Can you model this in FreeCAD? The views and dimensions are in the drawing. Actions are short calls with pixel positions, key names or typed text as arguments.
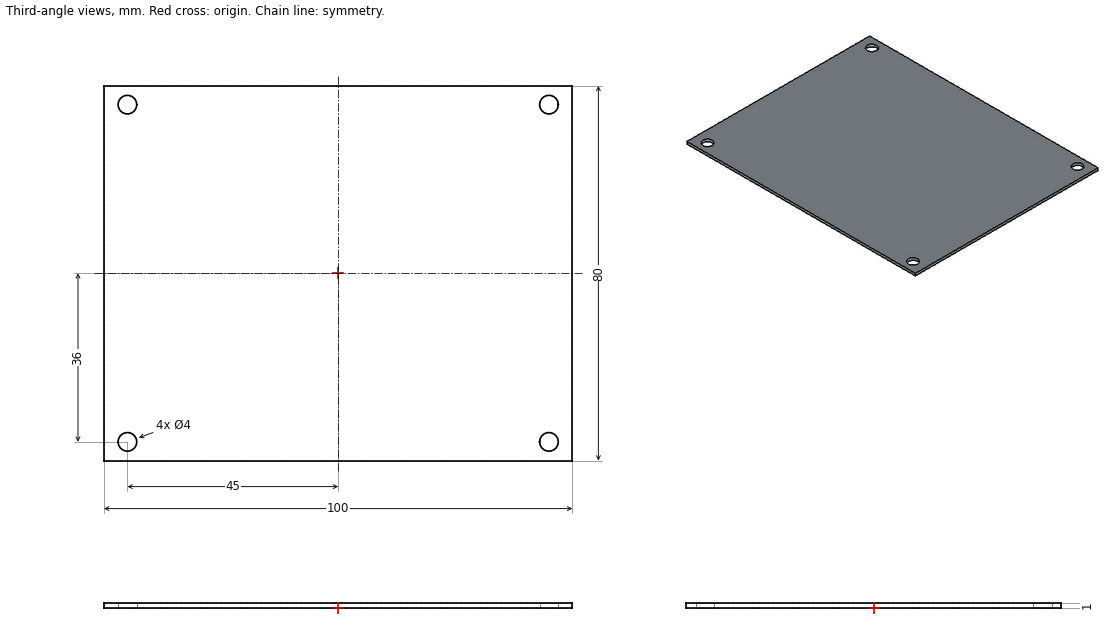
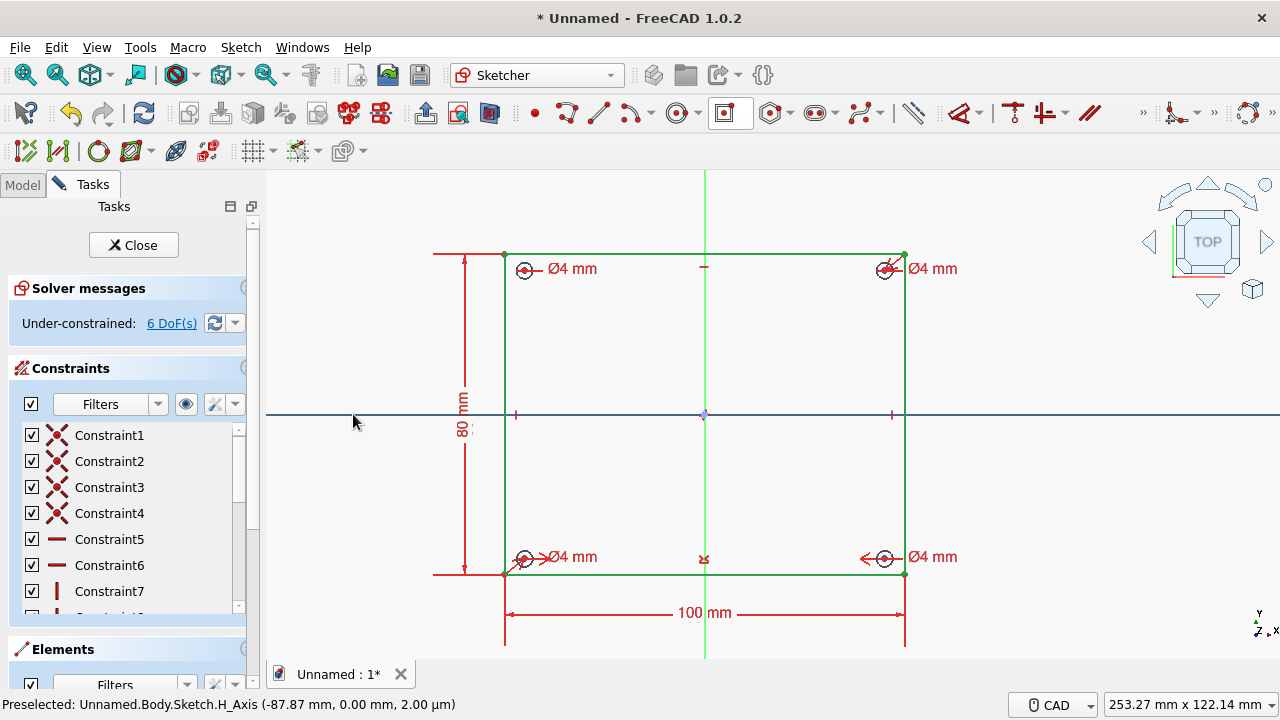
key(s)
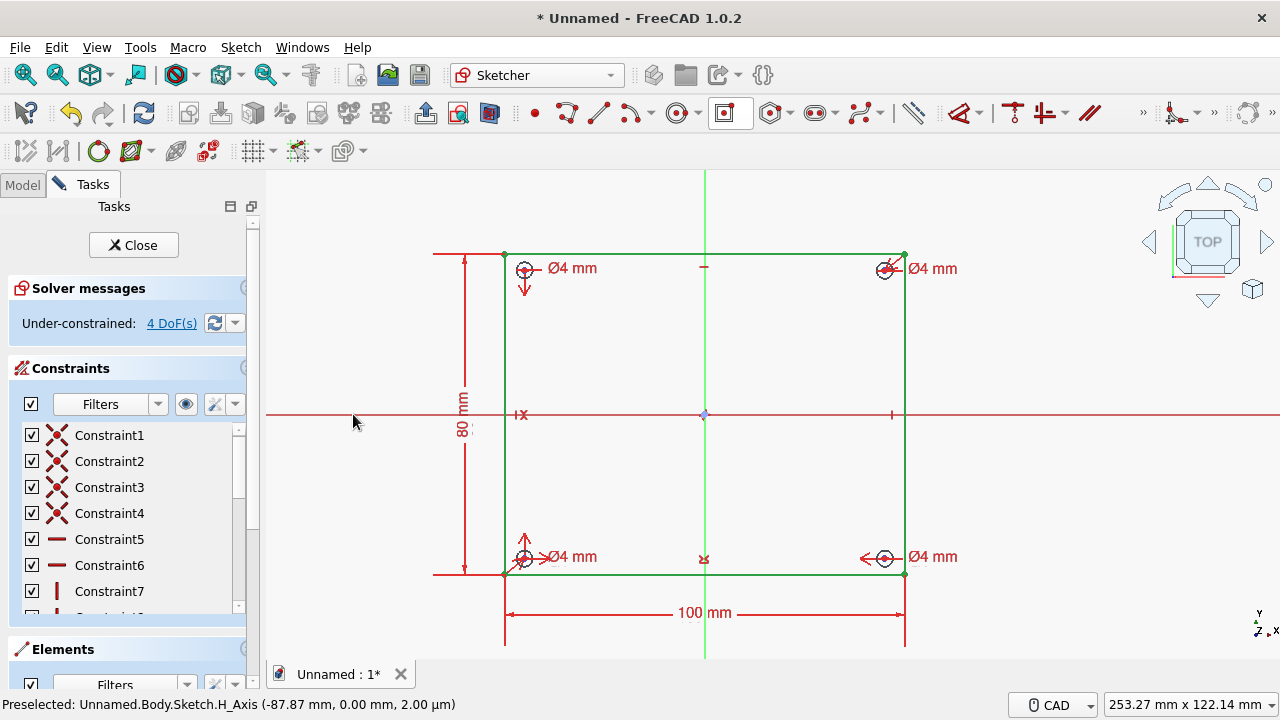
click(885, 559)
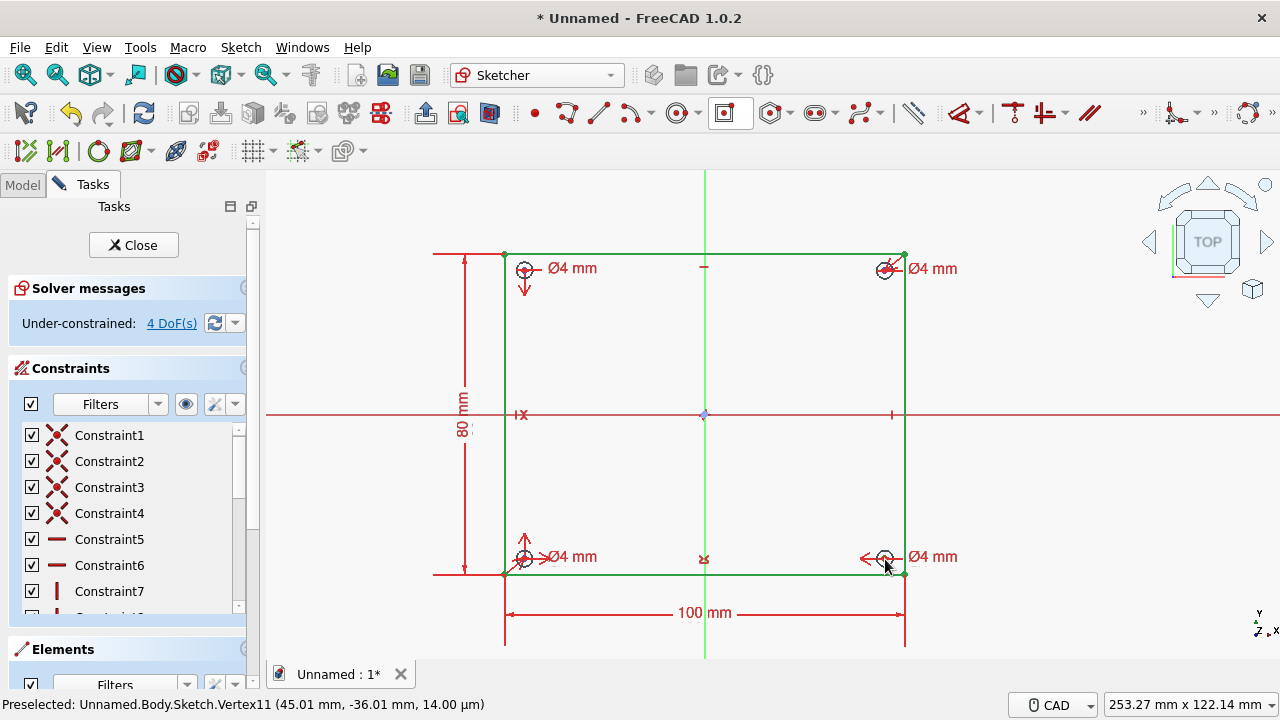
click(885, 271)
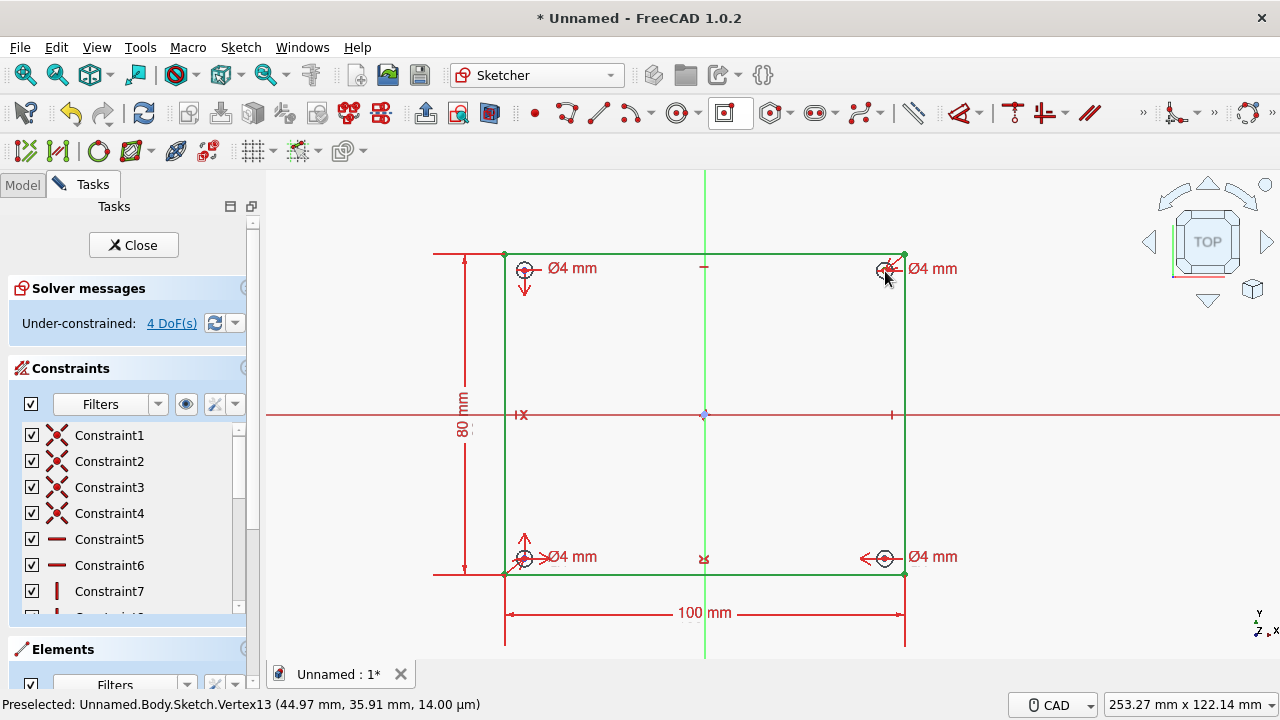
click(353, 414)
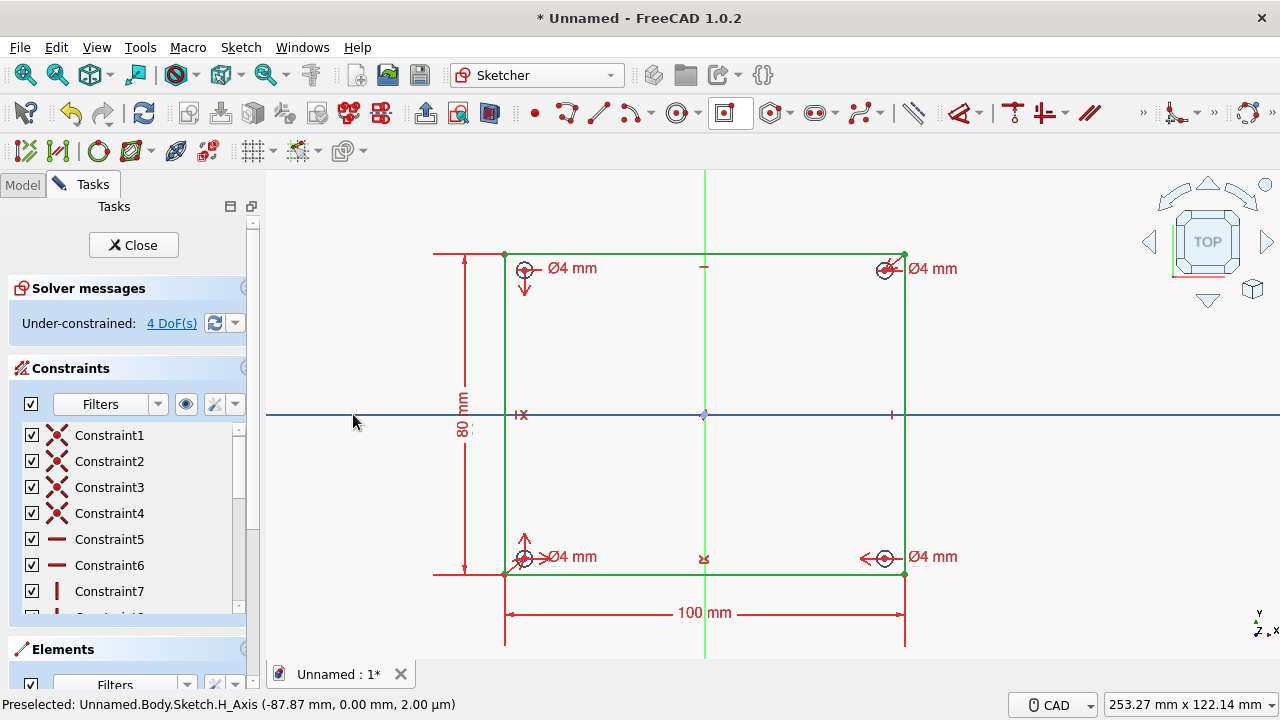
key(s)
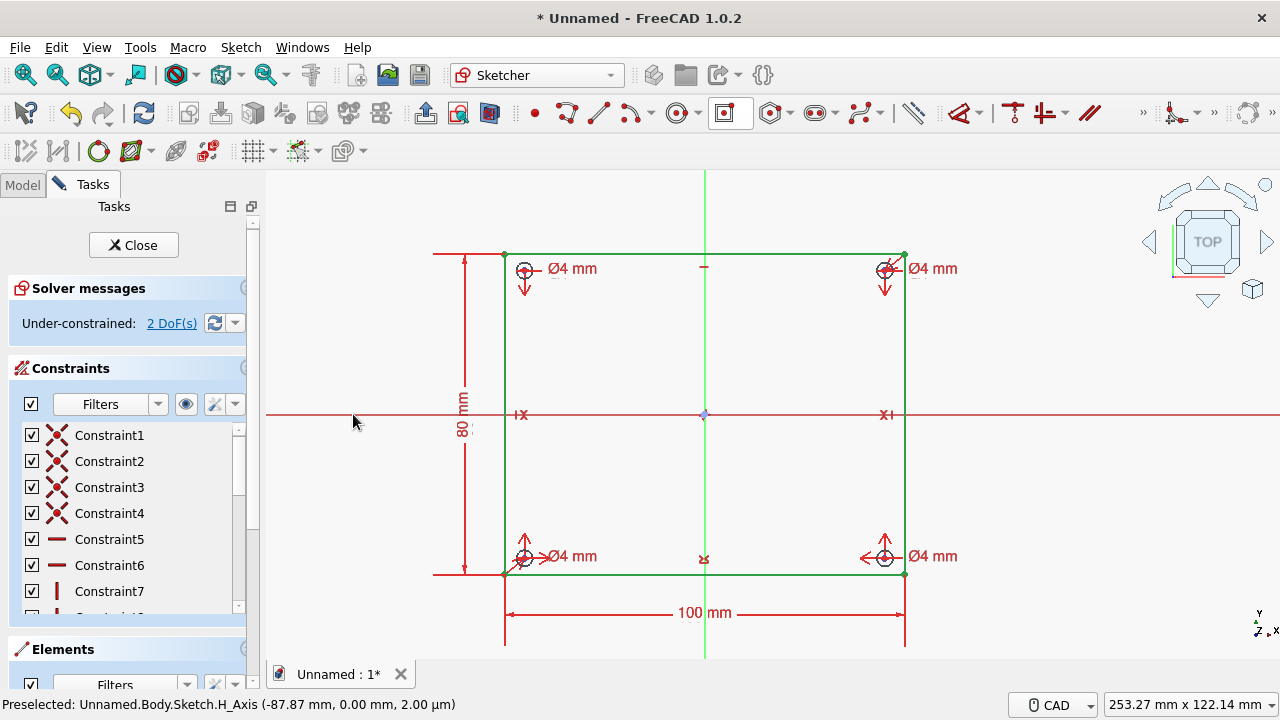
click(525, 558)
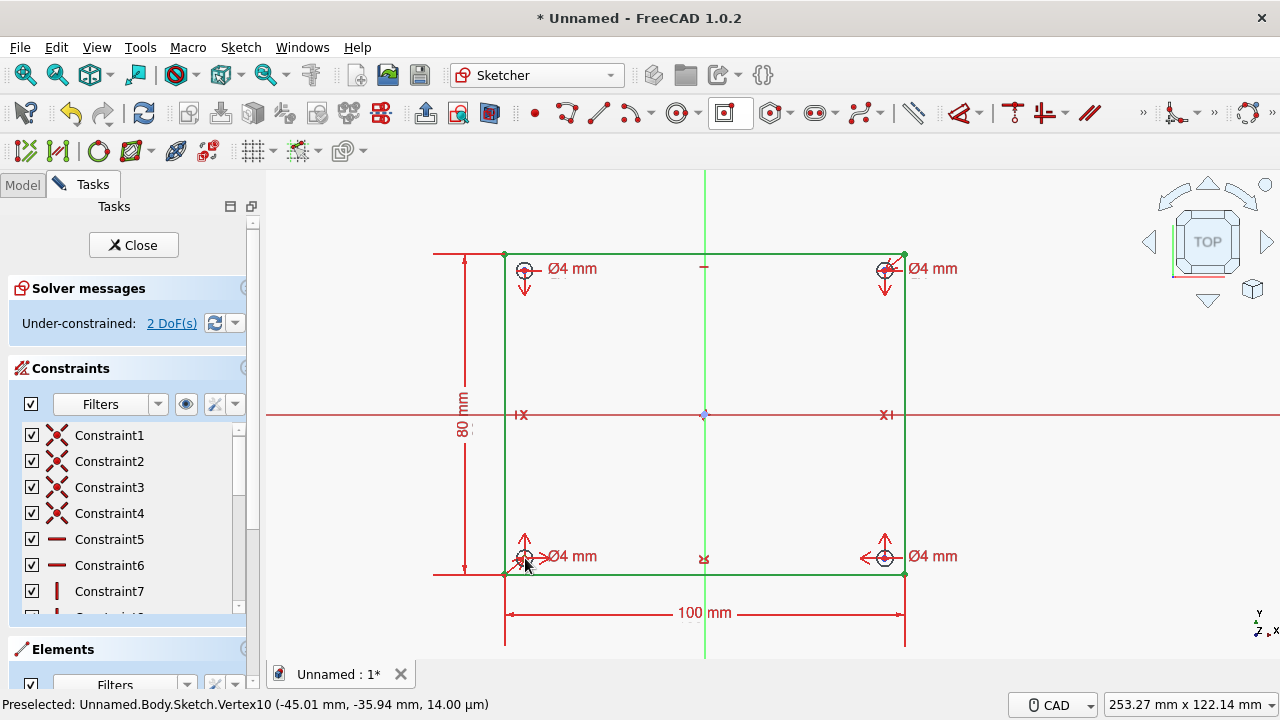
click(982, 114)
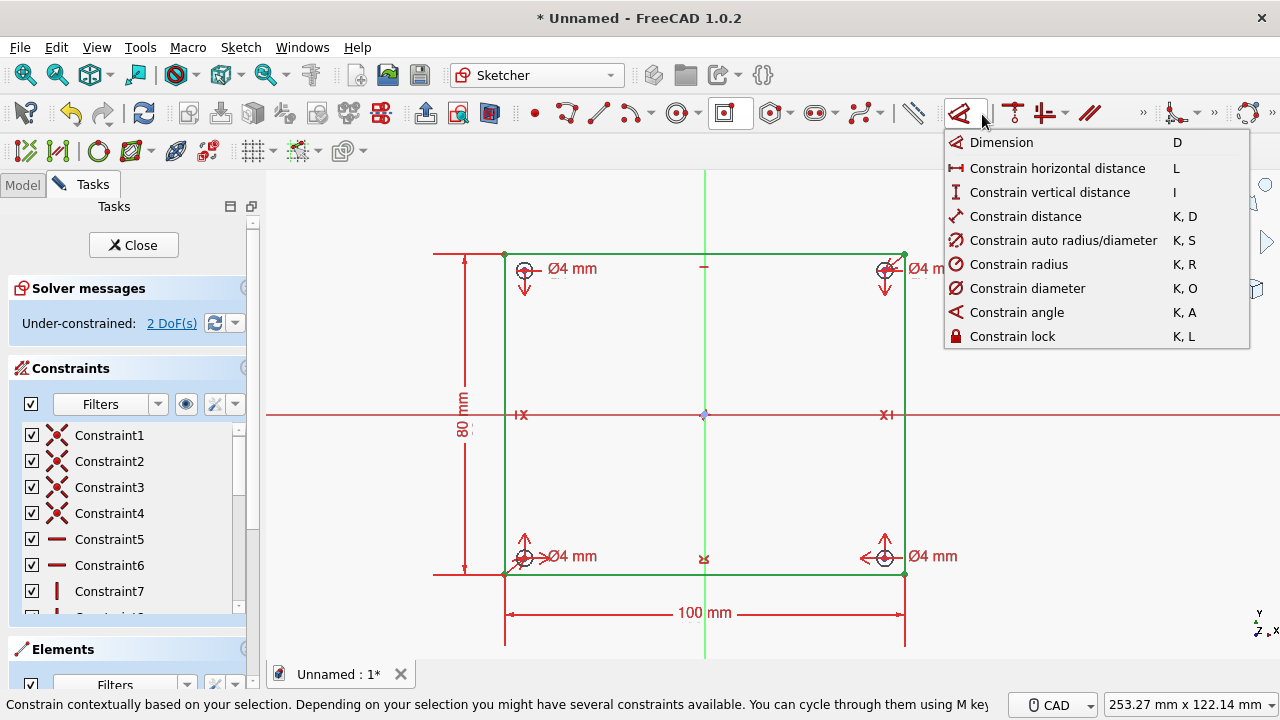
click(1097, 168)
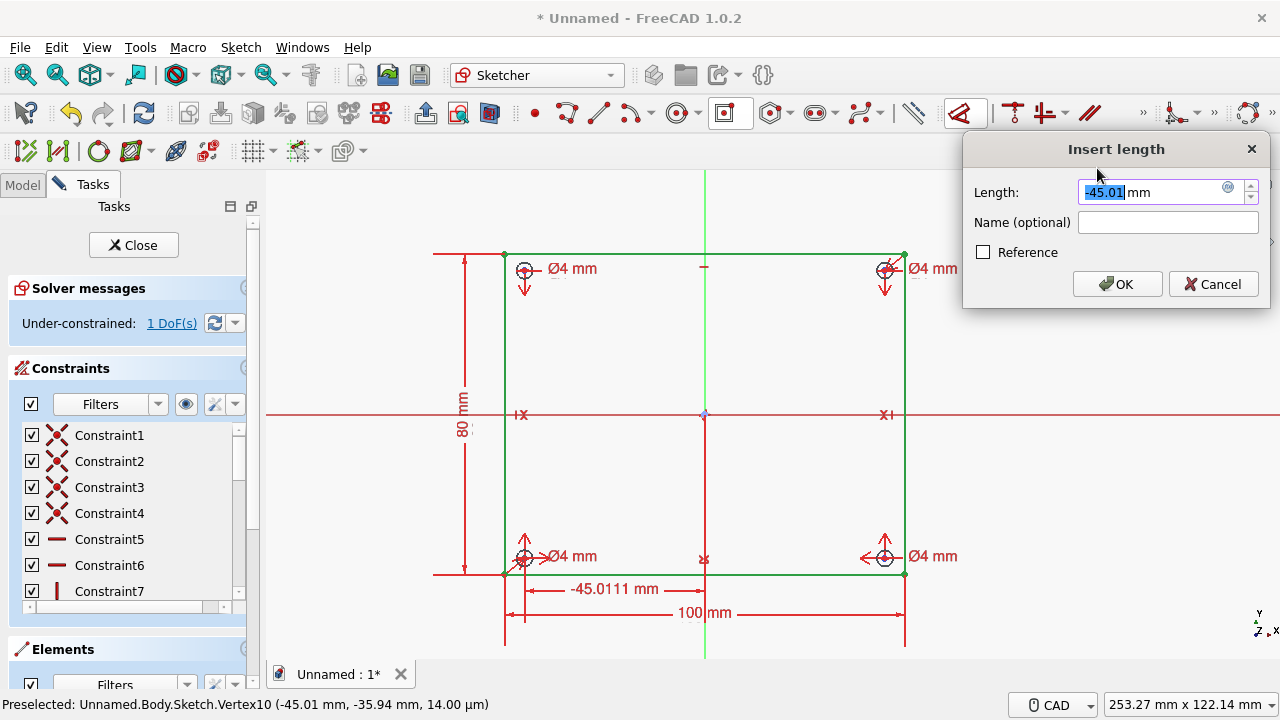
text(-45)
key(Return)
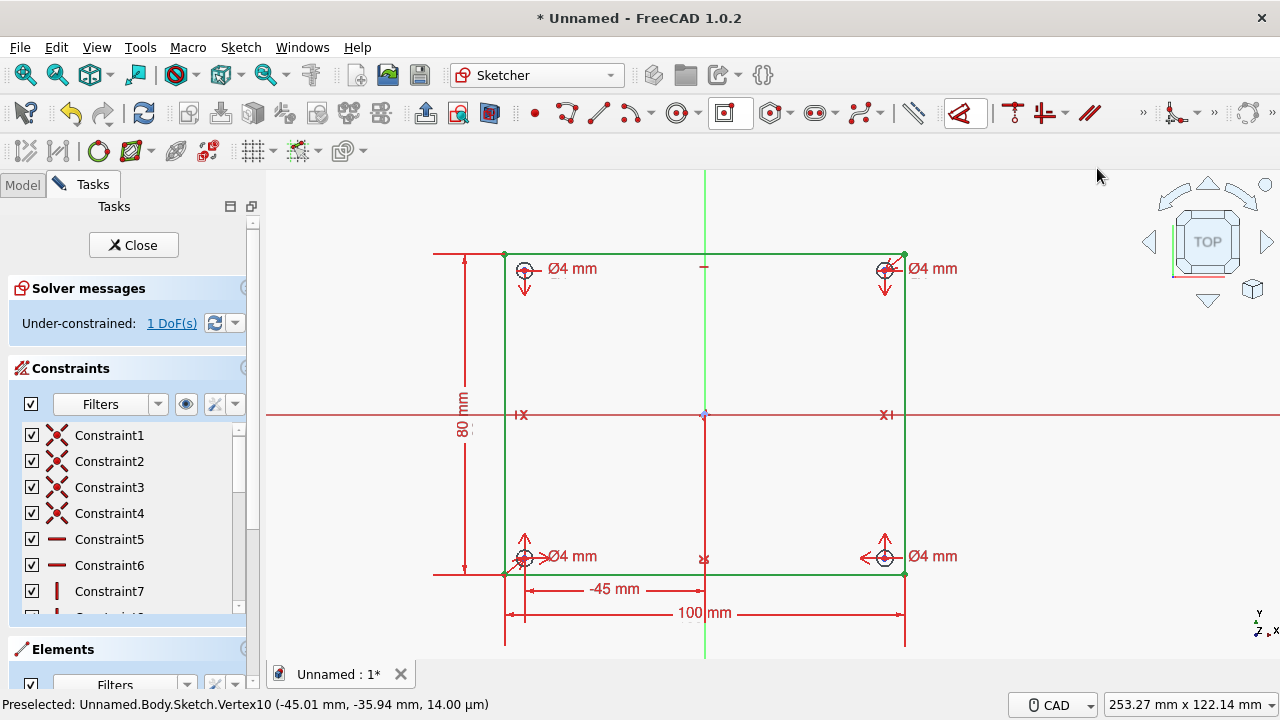
click(525, 558)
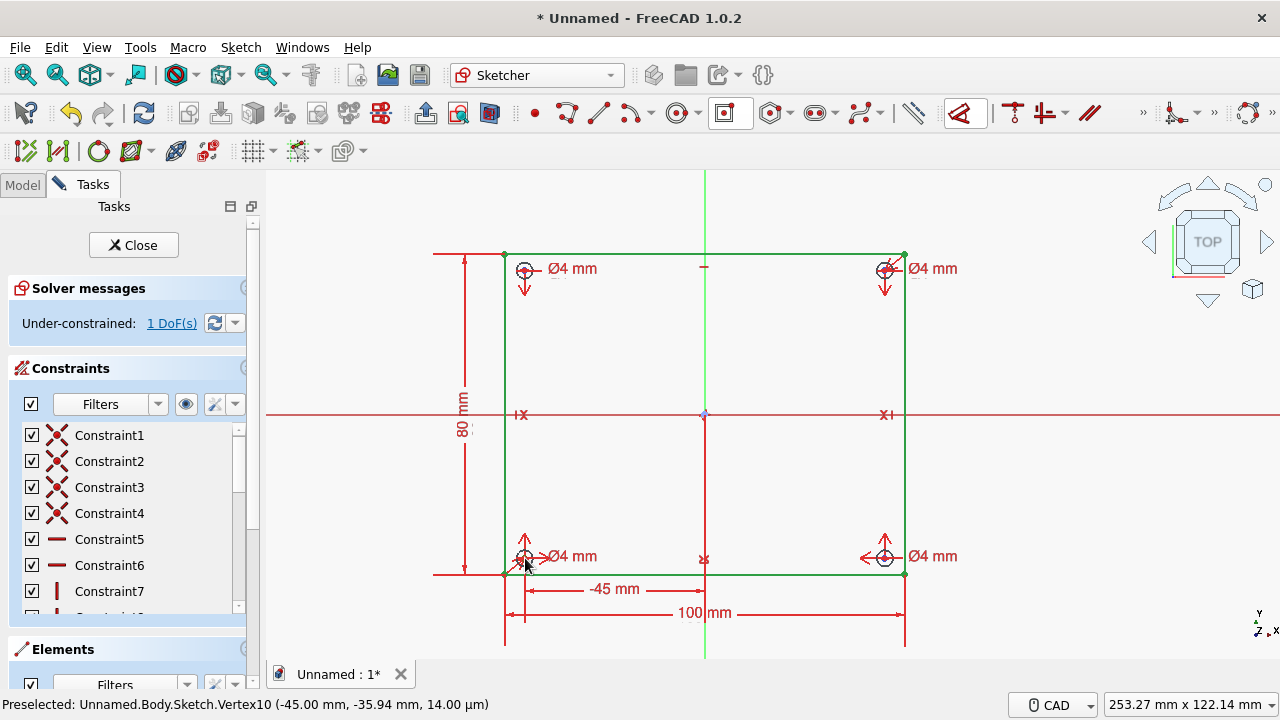
key(i)